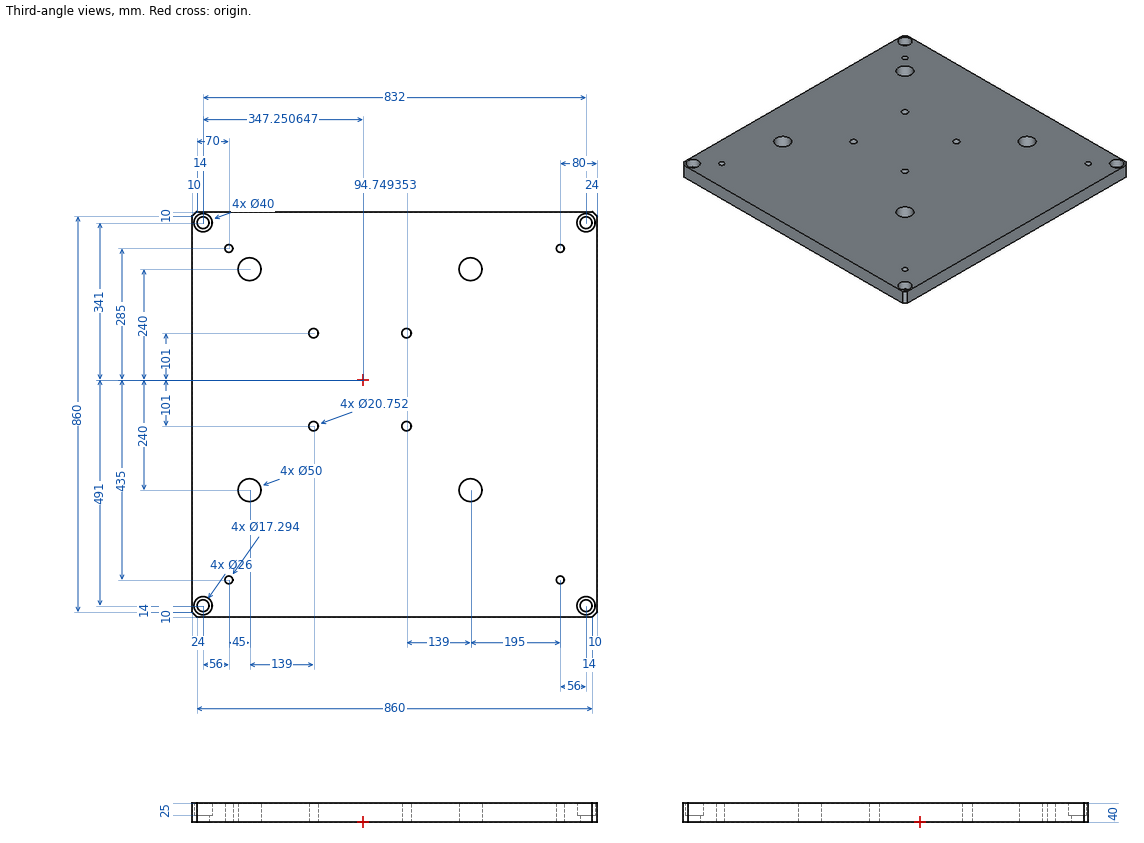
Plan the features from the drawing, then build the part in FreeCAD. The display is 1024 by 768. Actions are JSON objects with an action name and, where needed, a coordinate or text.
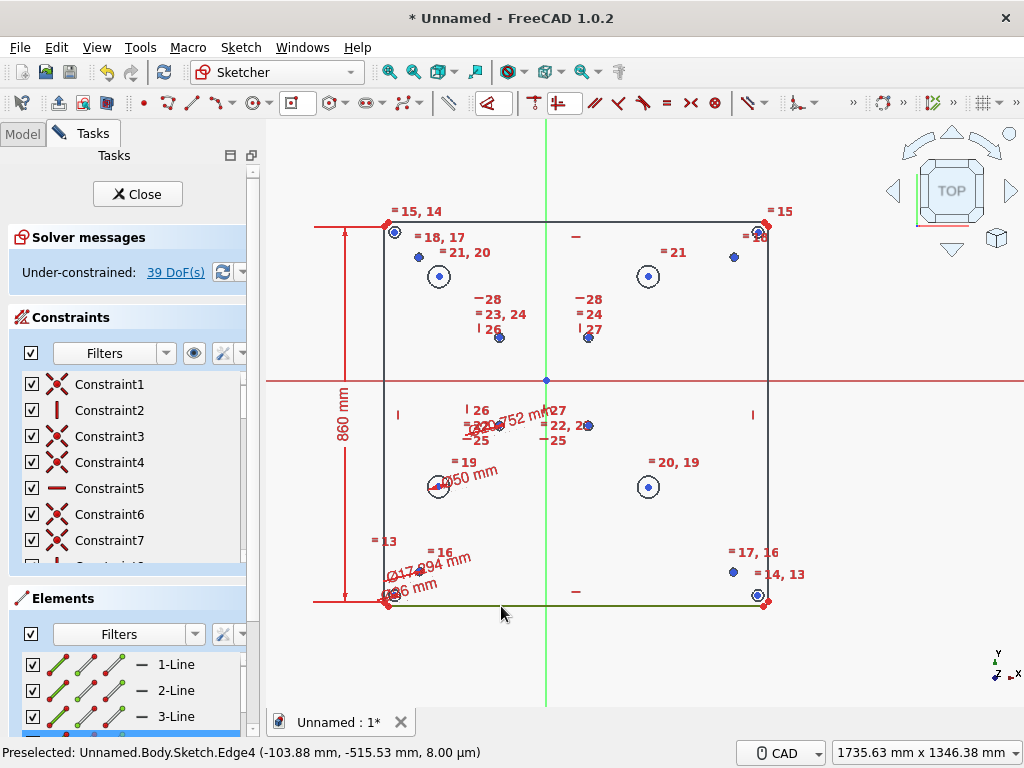
{"action": "key", "text": "l"}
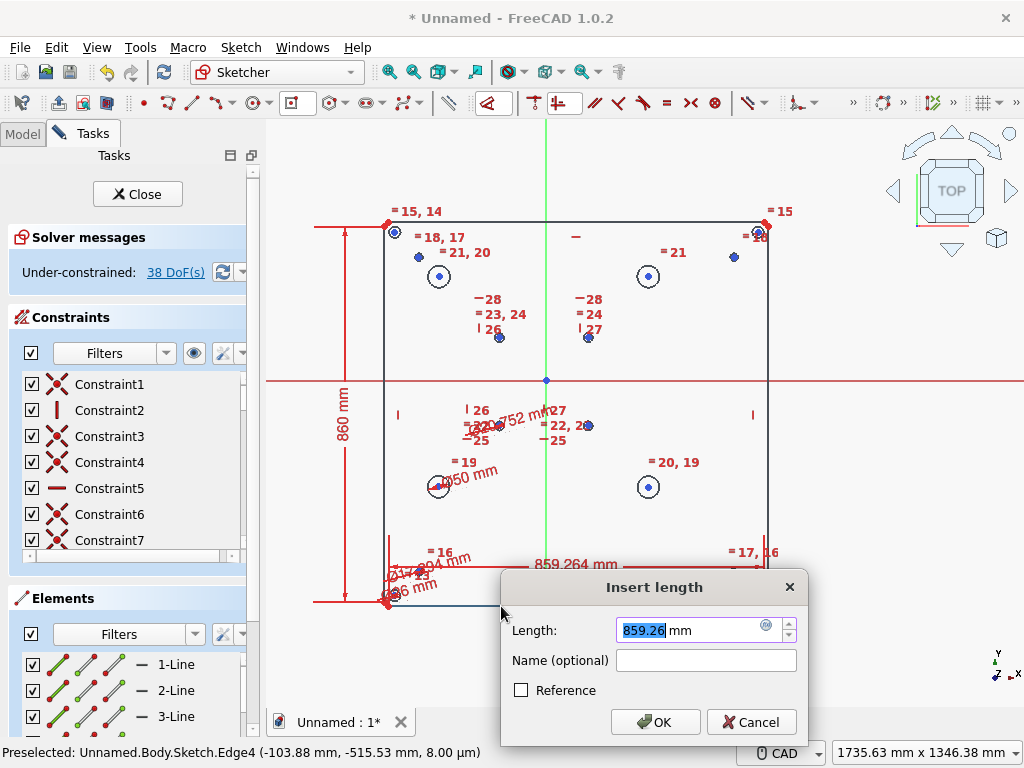
{"action": "type", "text": "860"}
{"action": "key", "text": "Return"}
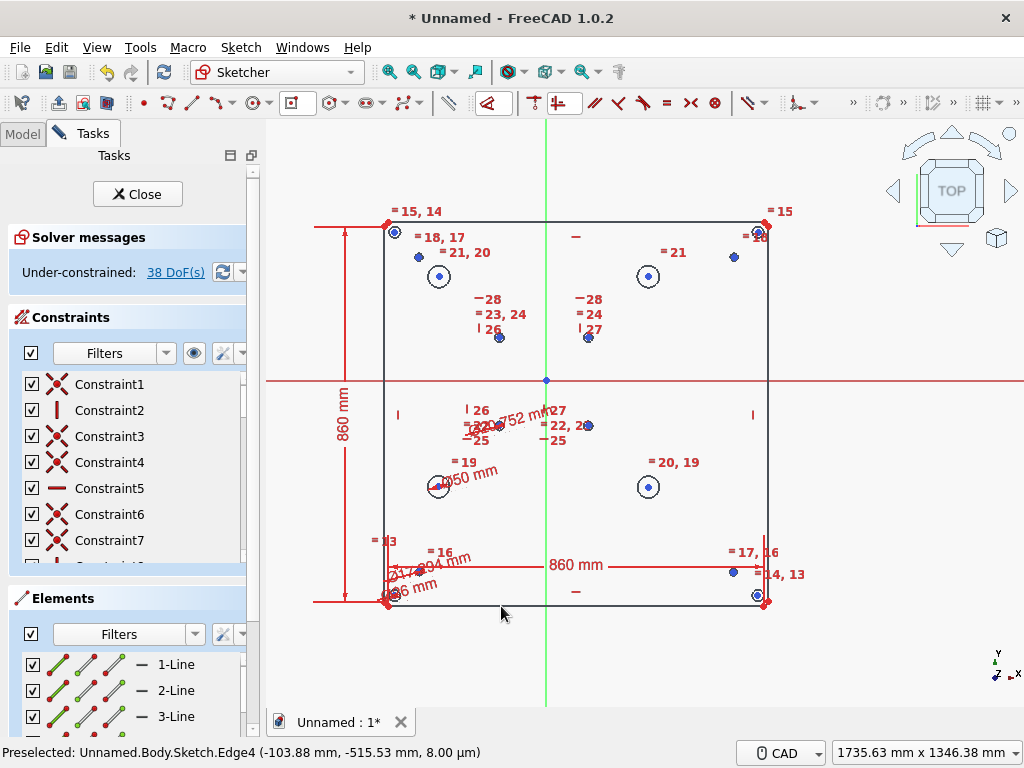
{"action": "left_click", "coordinate": [768, 489]}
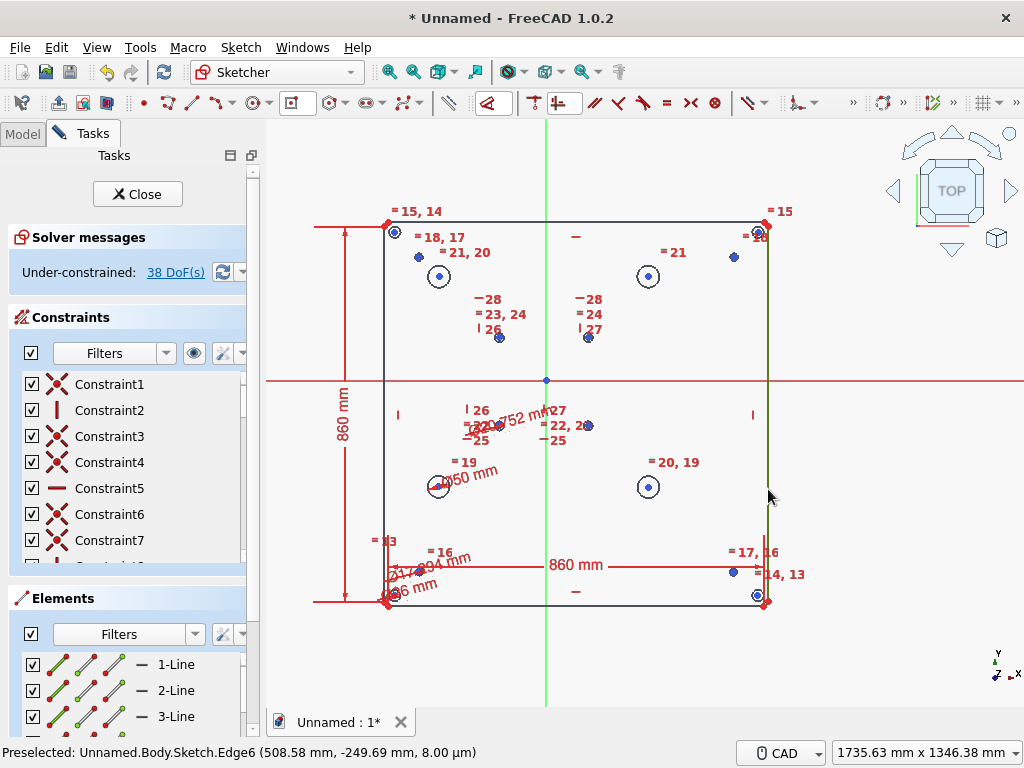
{"action": "key", "text": "i"}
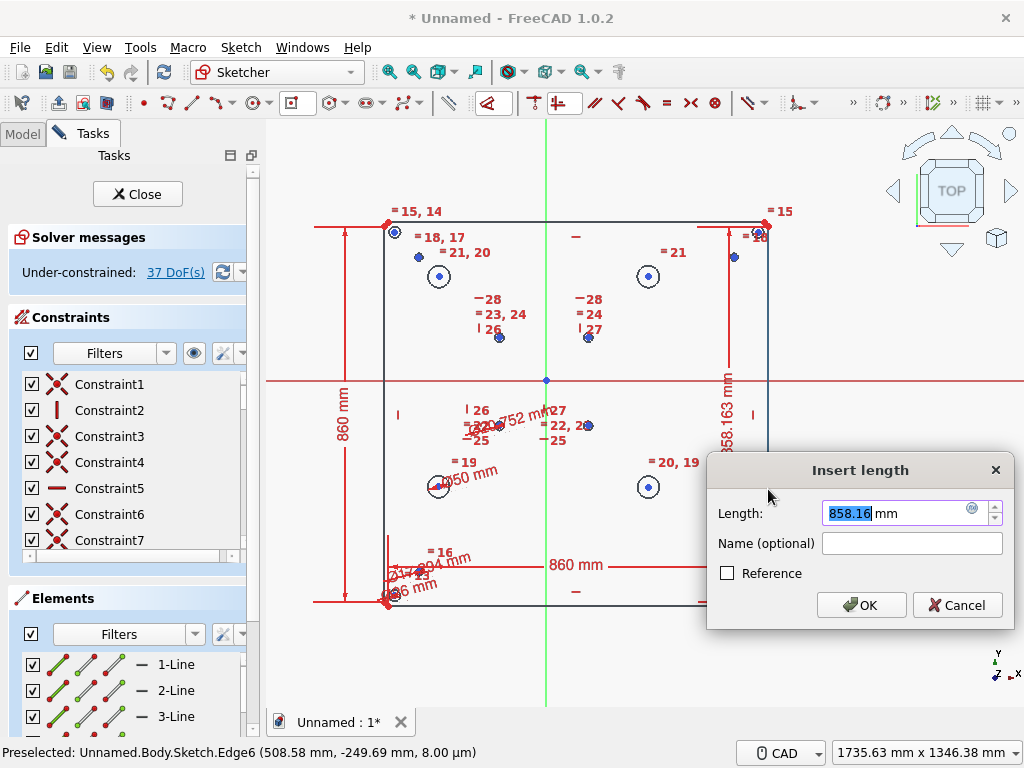
{"action": "type", "text": "860"}
{"action": "key", "text": "Return"}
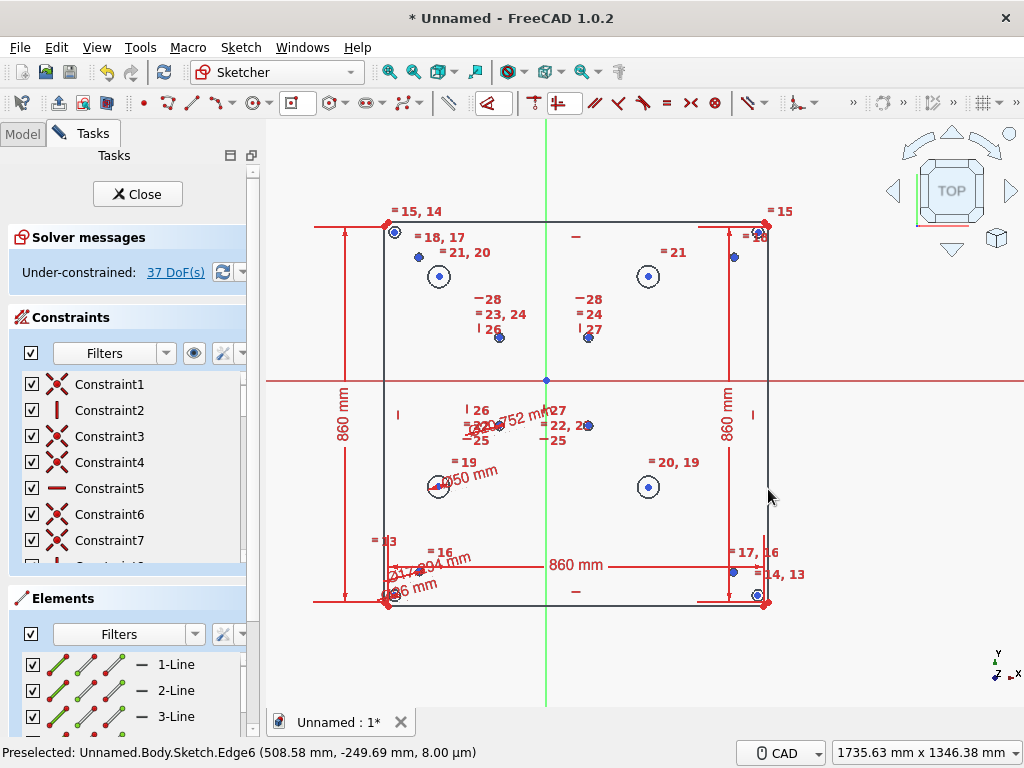
{"action": "left_click", "coordinate": [651, 222]}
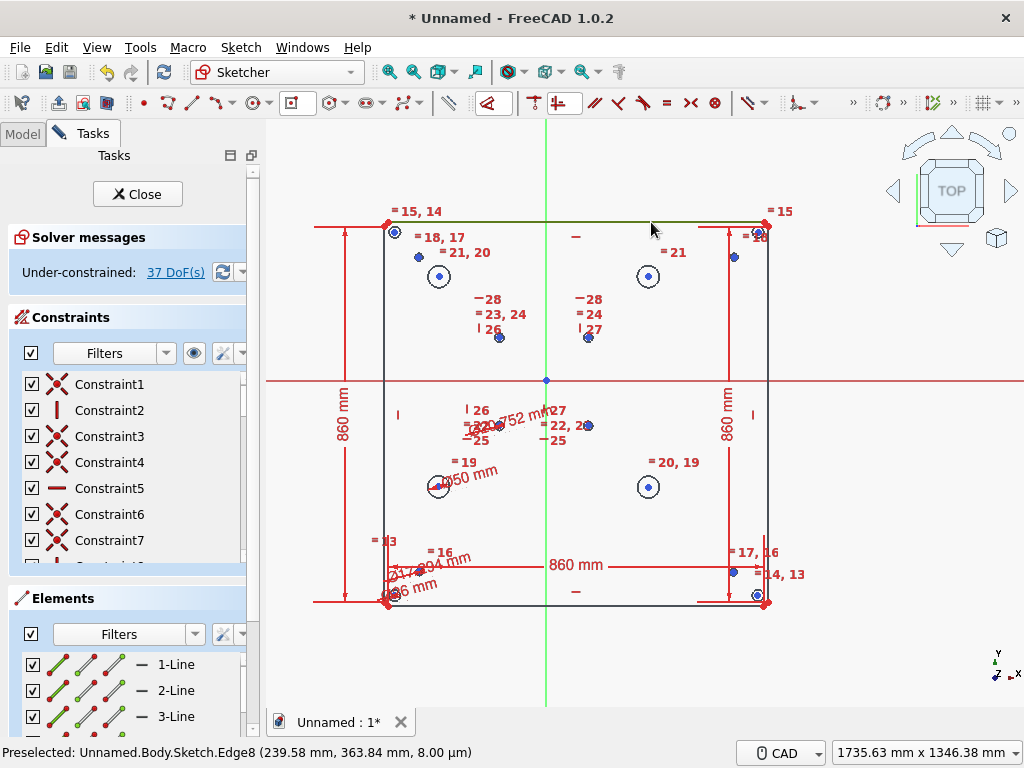
{"action": "key", "text": "l"}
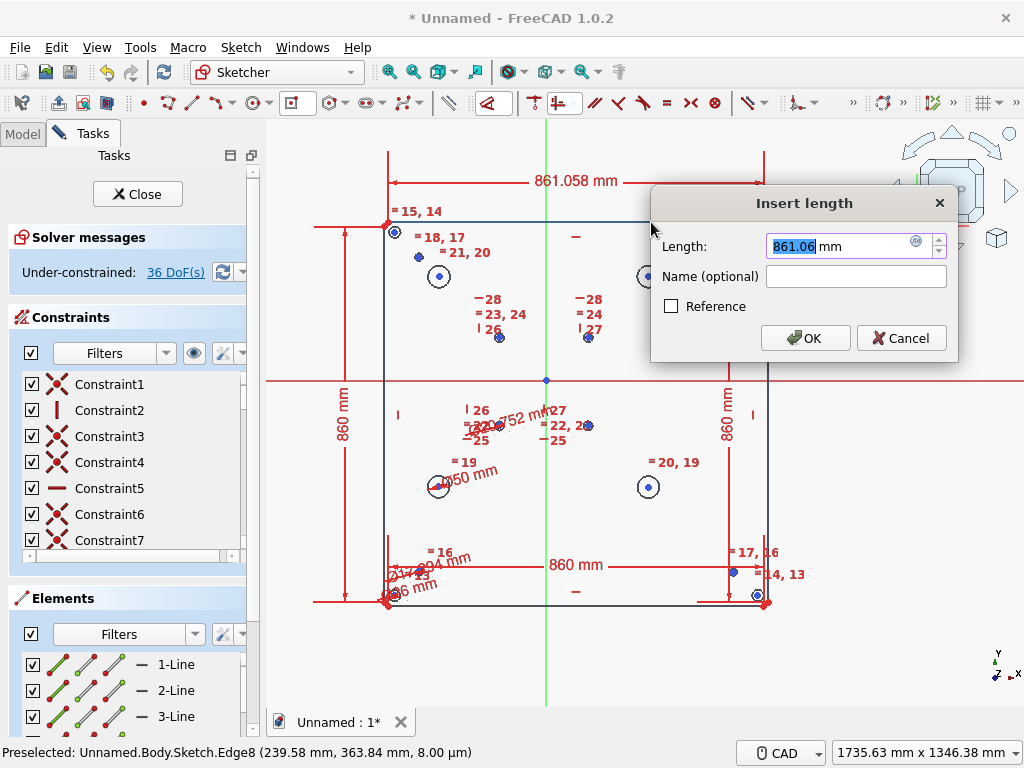
{"action": "type", "text": "860"}
{"action": "key", "text": "Return"}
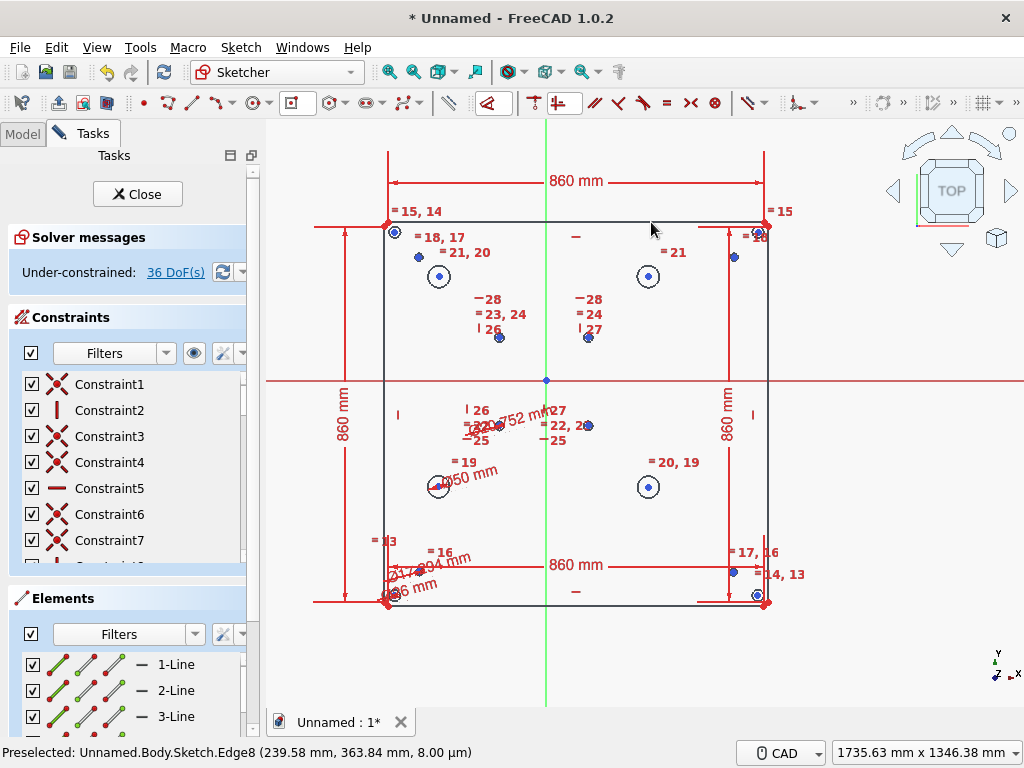
{"action": "scroll", "coordinate": [386, 224], "scroll_direction": "up", "scroll_amount": 12}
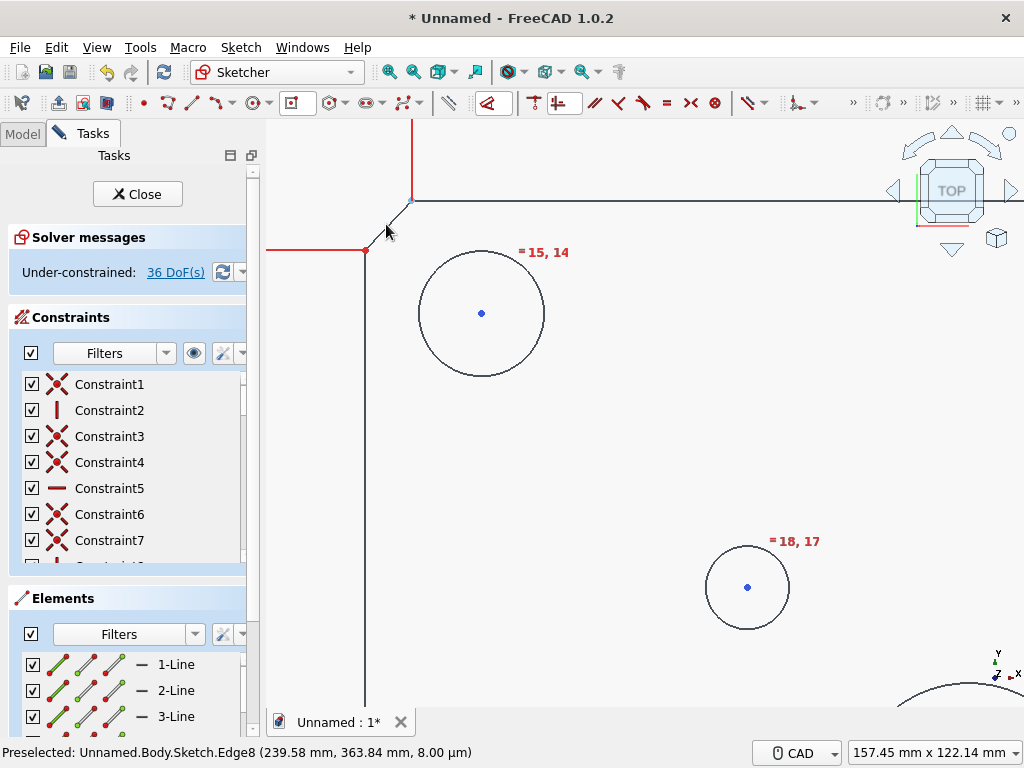
{"action": "left_click", "coordinate": [389, 226]}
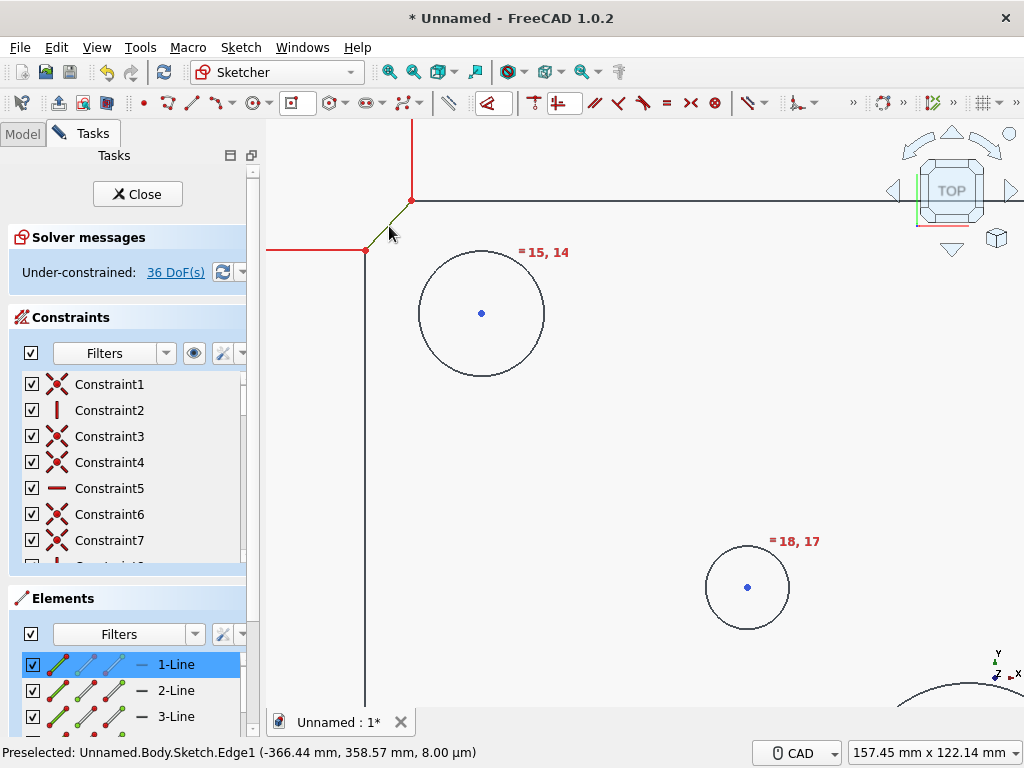
{"action": "key", "text": "l"}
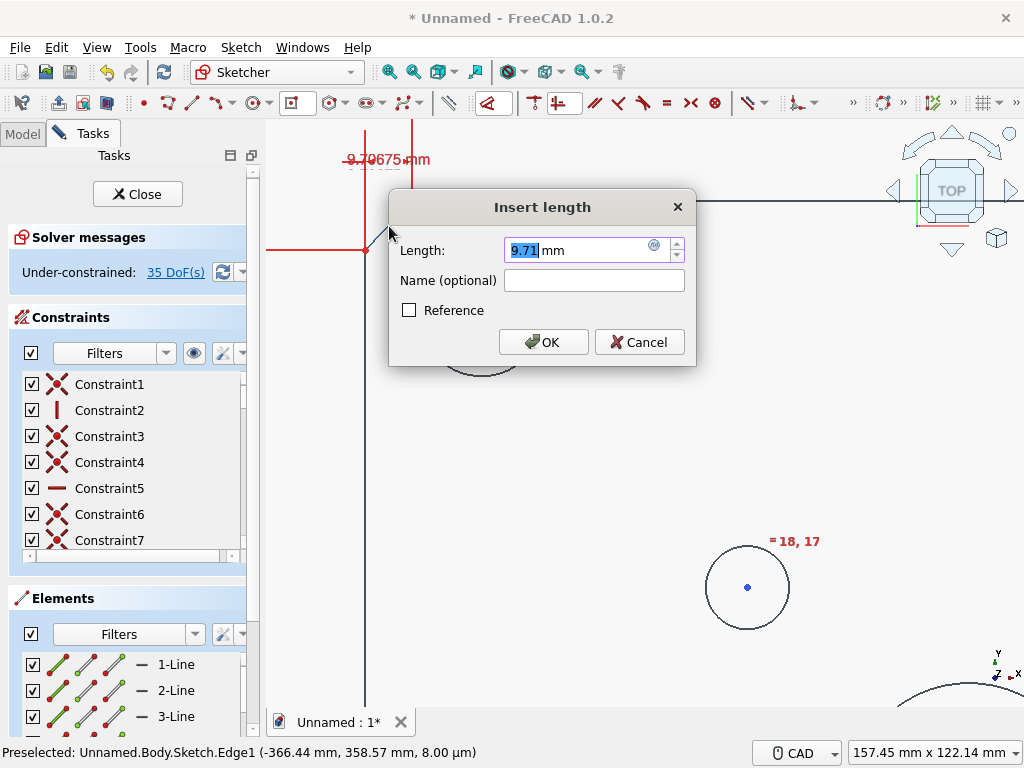
{"action": "type", "text": "10"}
{"action": "key", "text": "Return"}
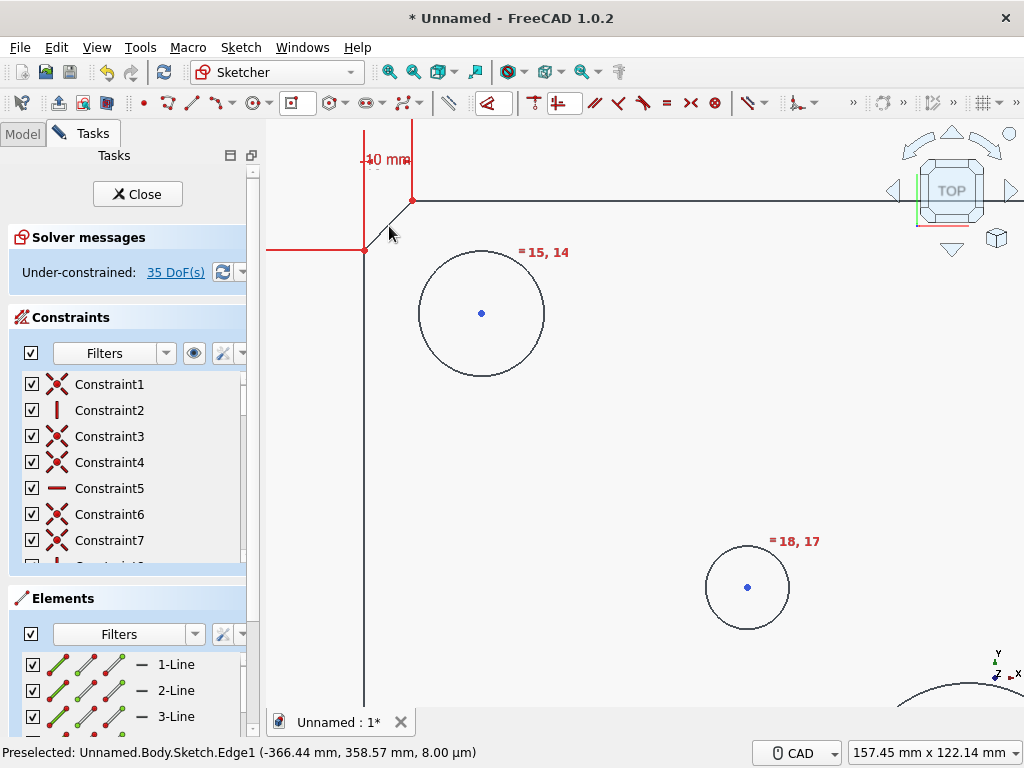
{"action": "left_click", "coordinate": [398, 216]}